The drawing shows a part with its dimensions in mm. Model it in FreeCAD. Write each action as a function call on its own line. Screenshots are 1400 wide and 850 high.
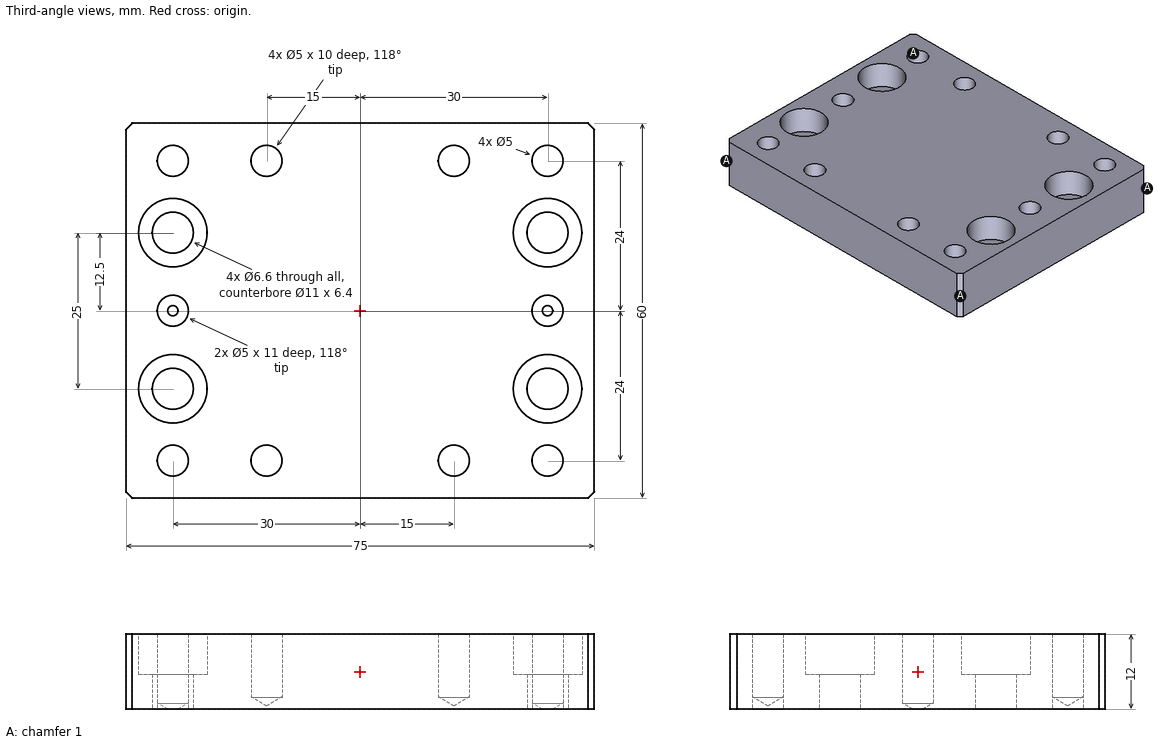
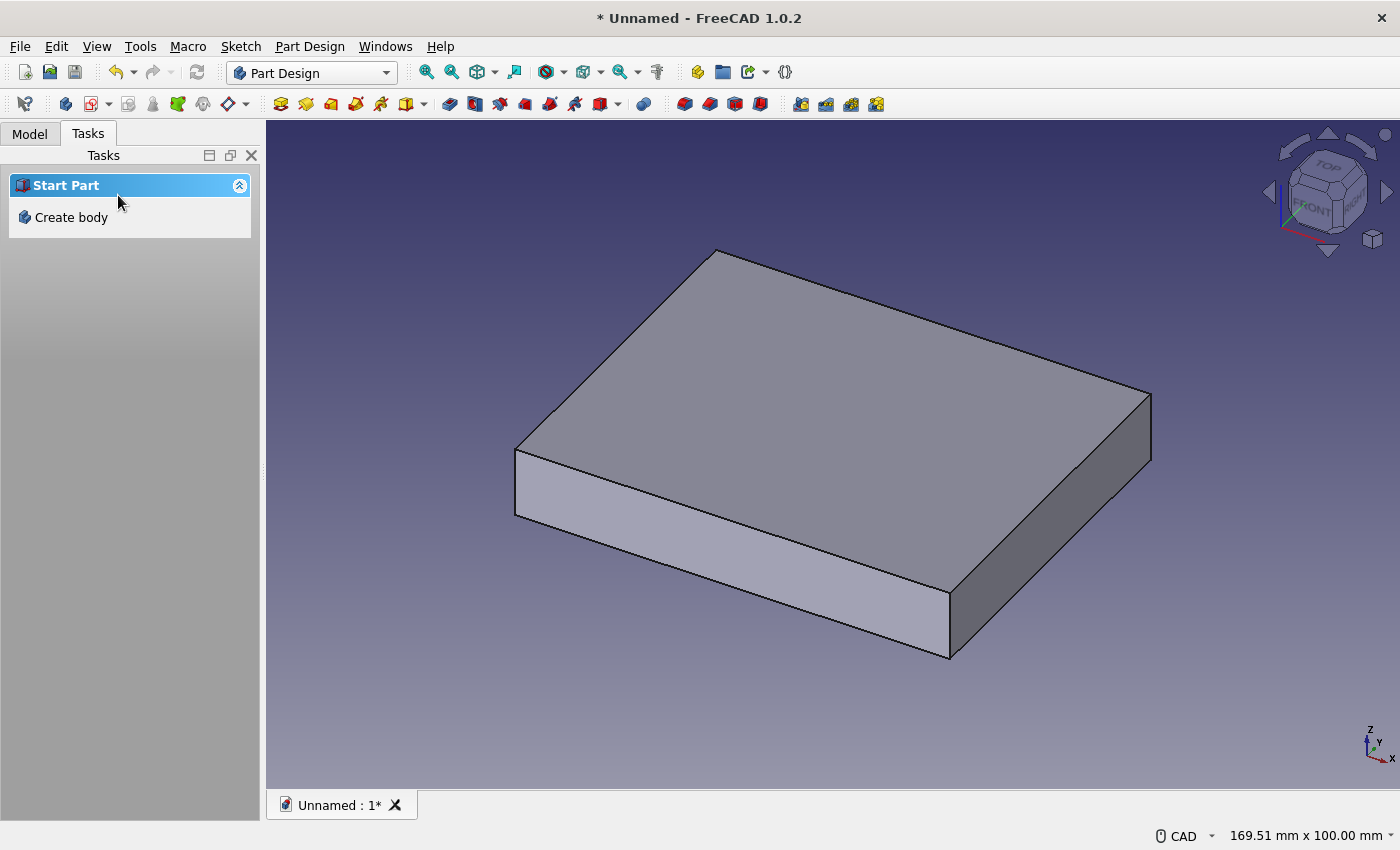
click(833, 421)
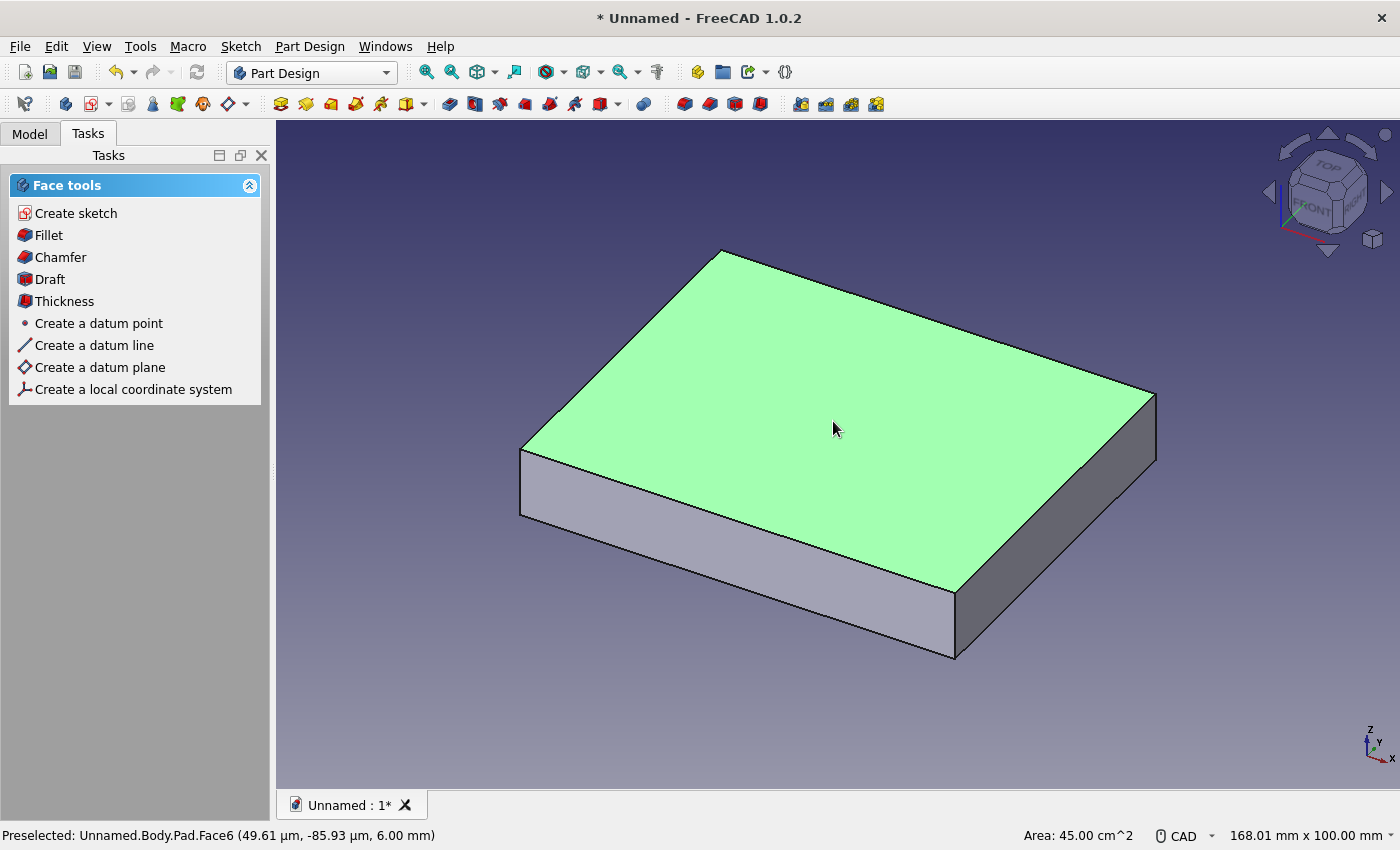
click(90, 104)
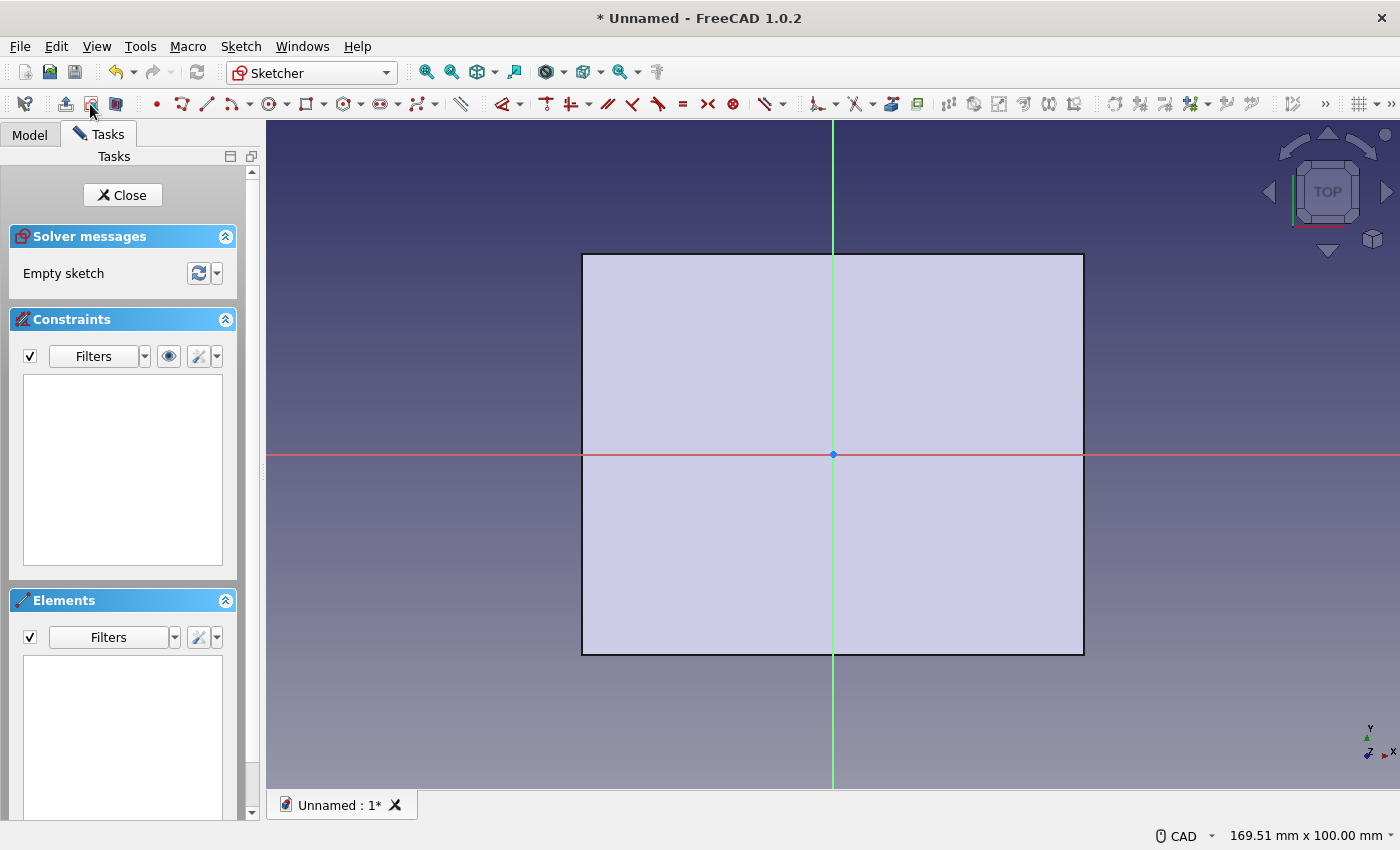
click(268, 104)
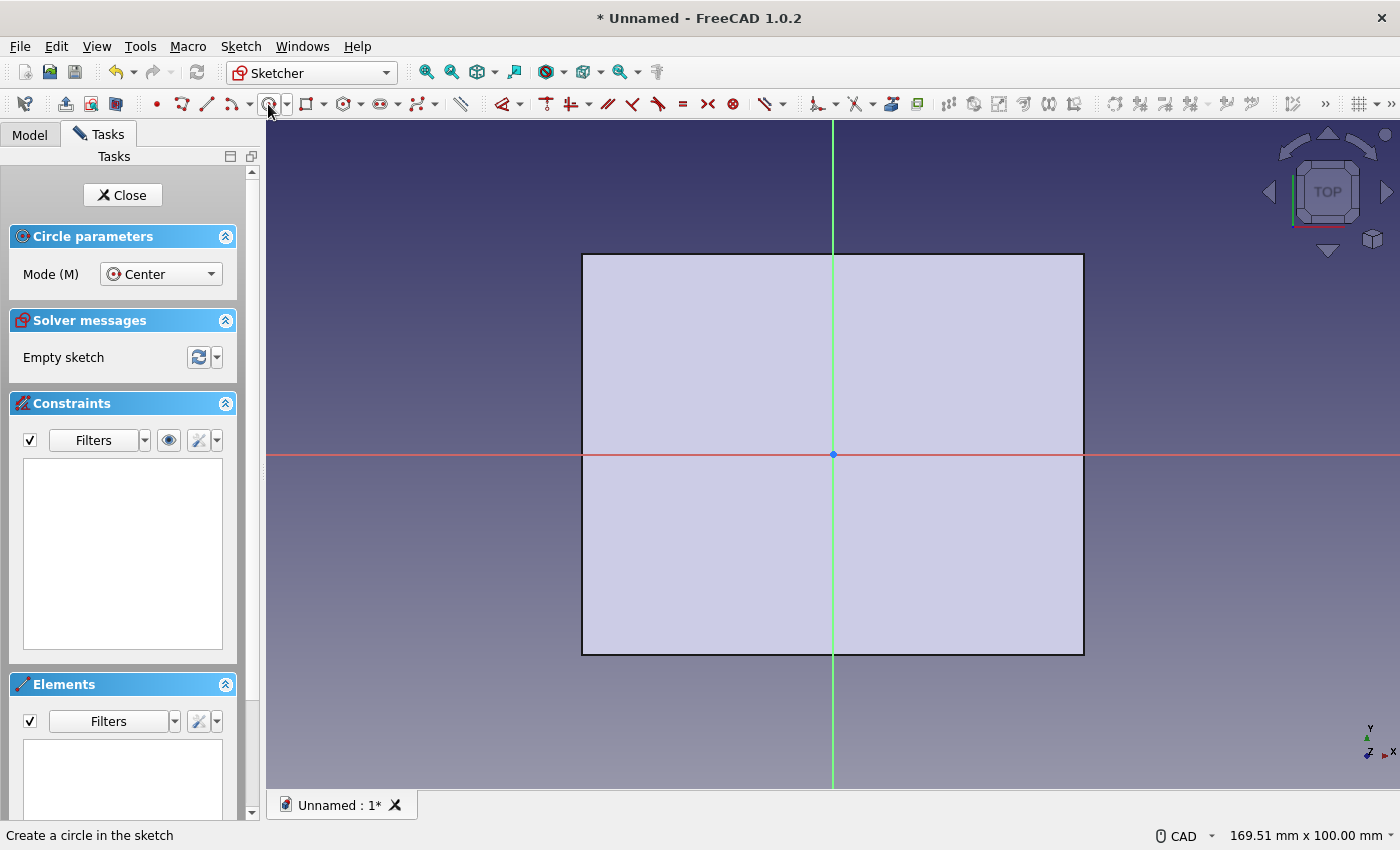
scroll(1034, 294, up, 2)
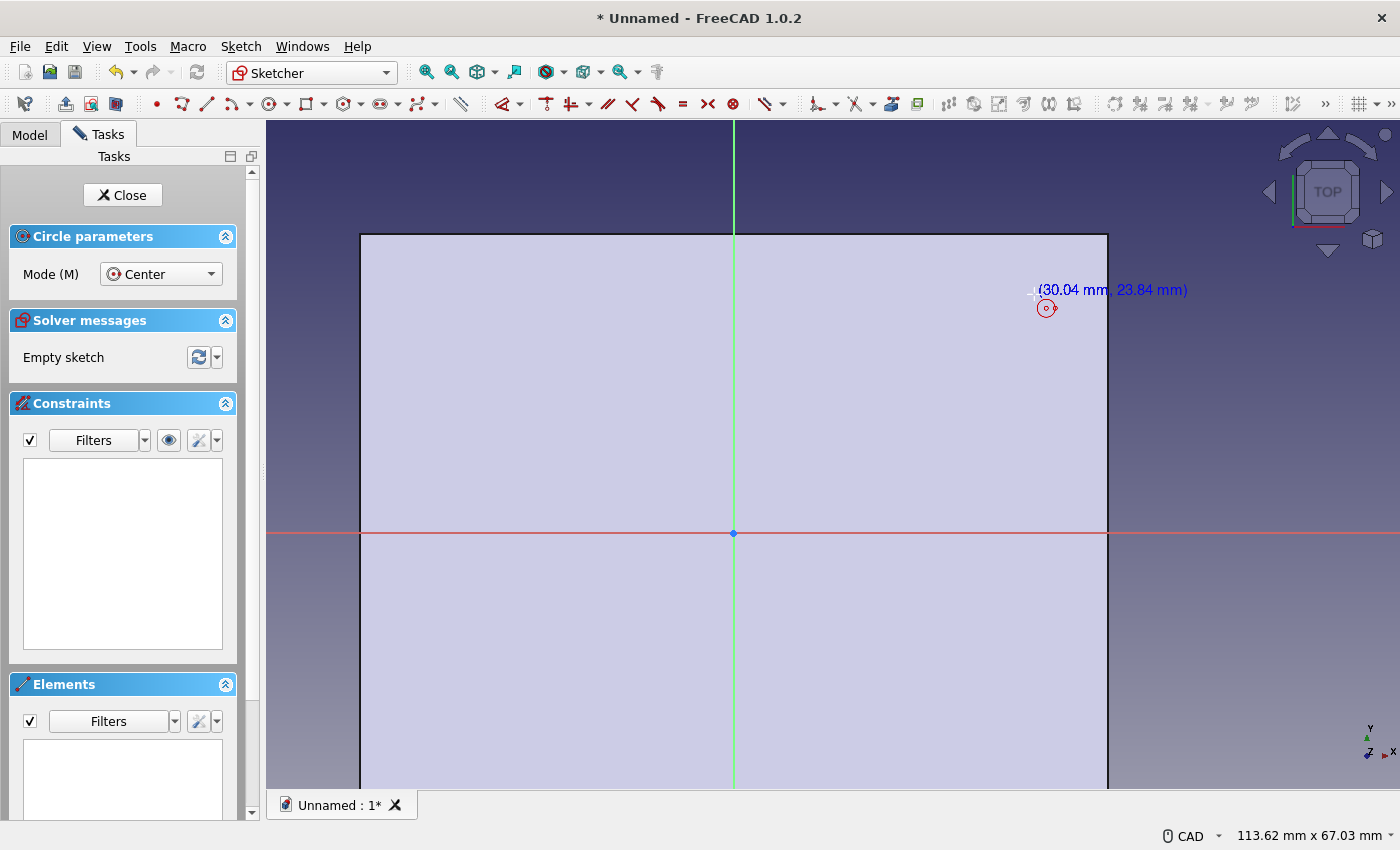
click(1033, 294)
click(1051, 276)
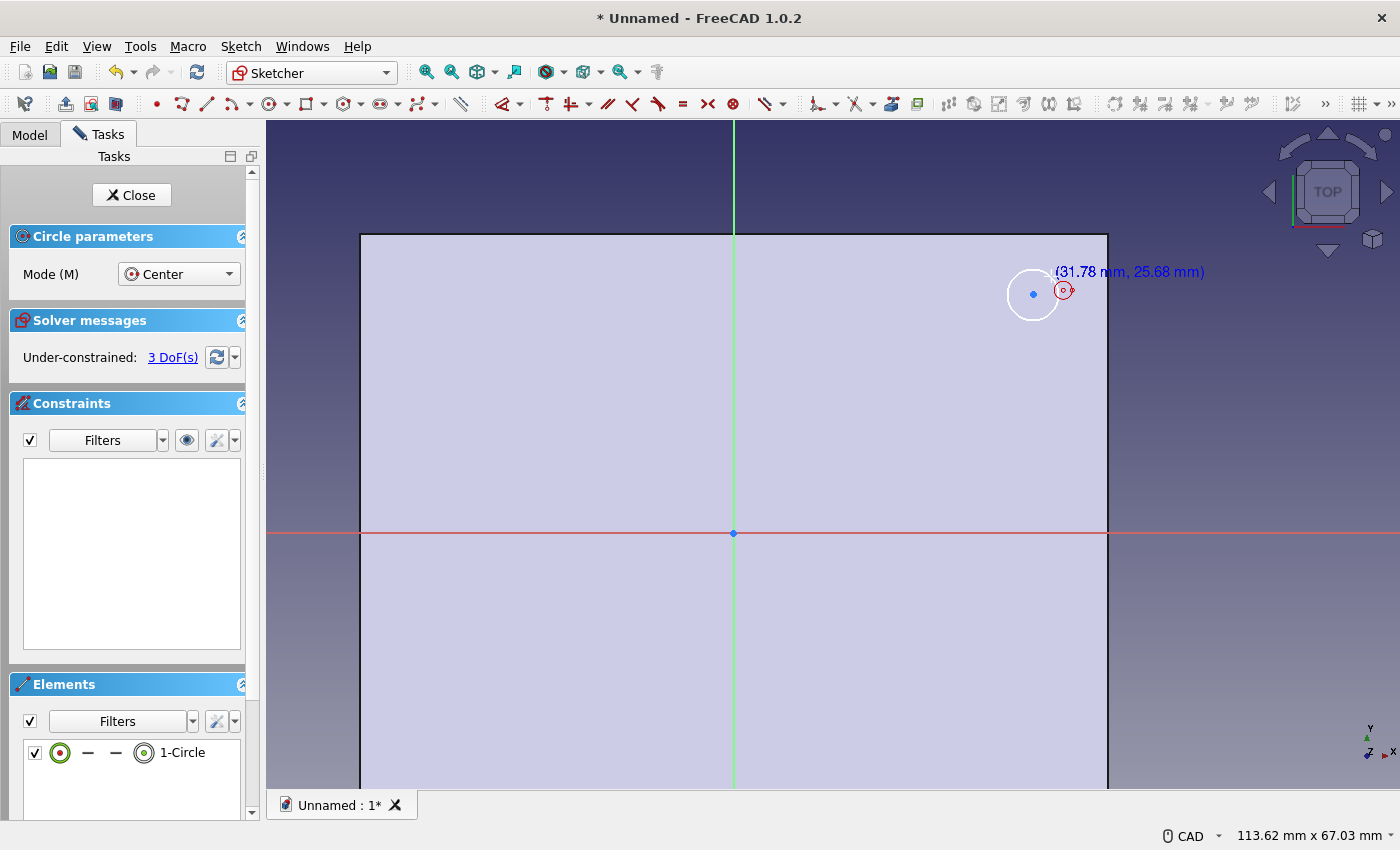
scroll(903, 148, down, 1)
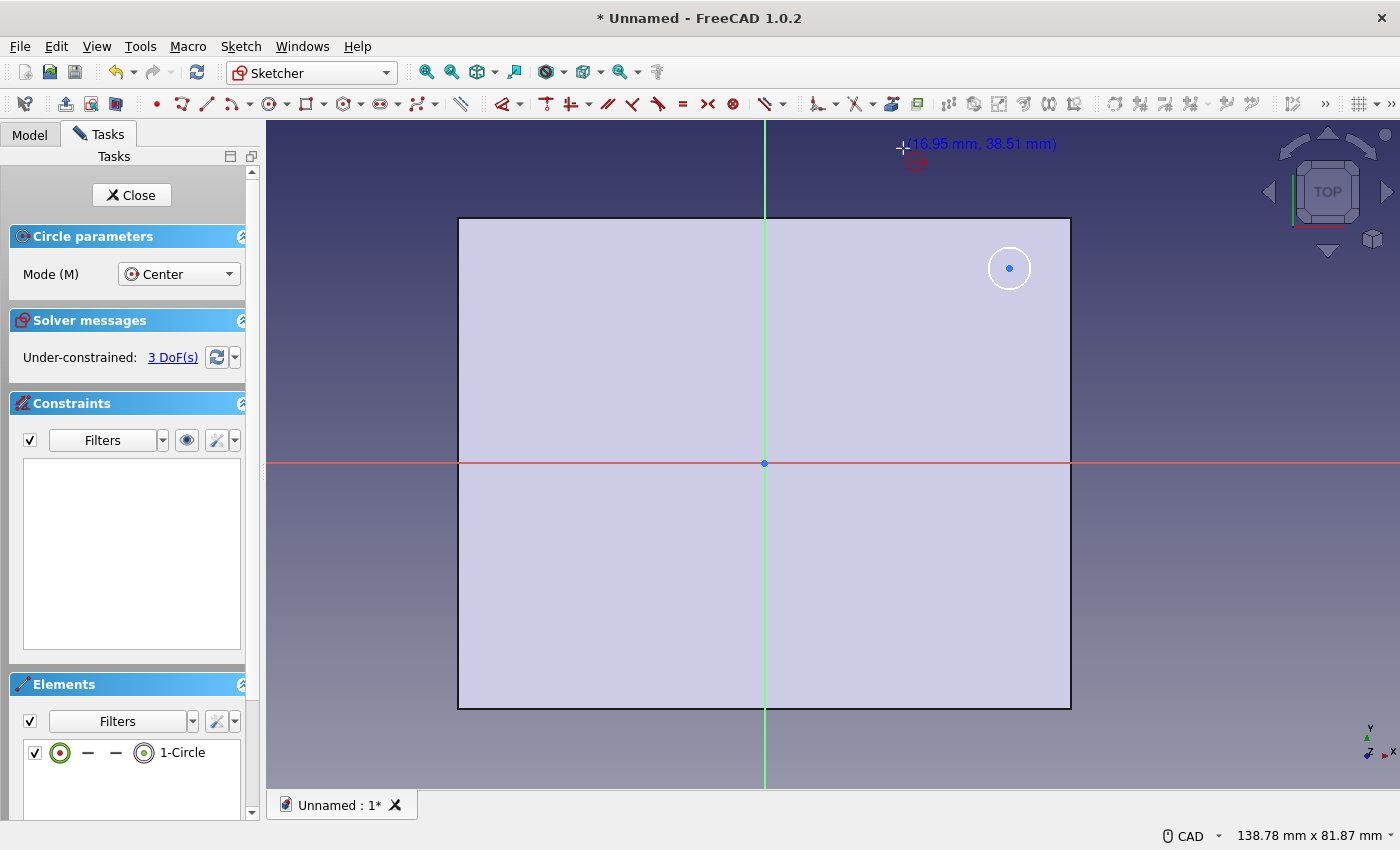
click(1010, 660)
click(1024, 645)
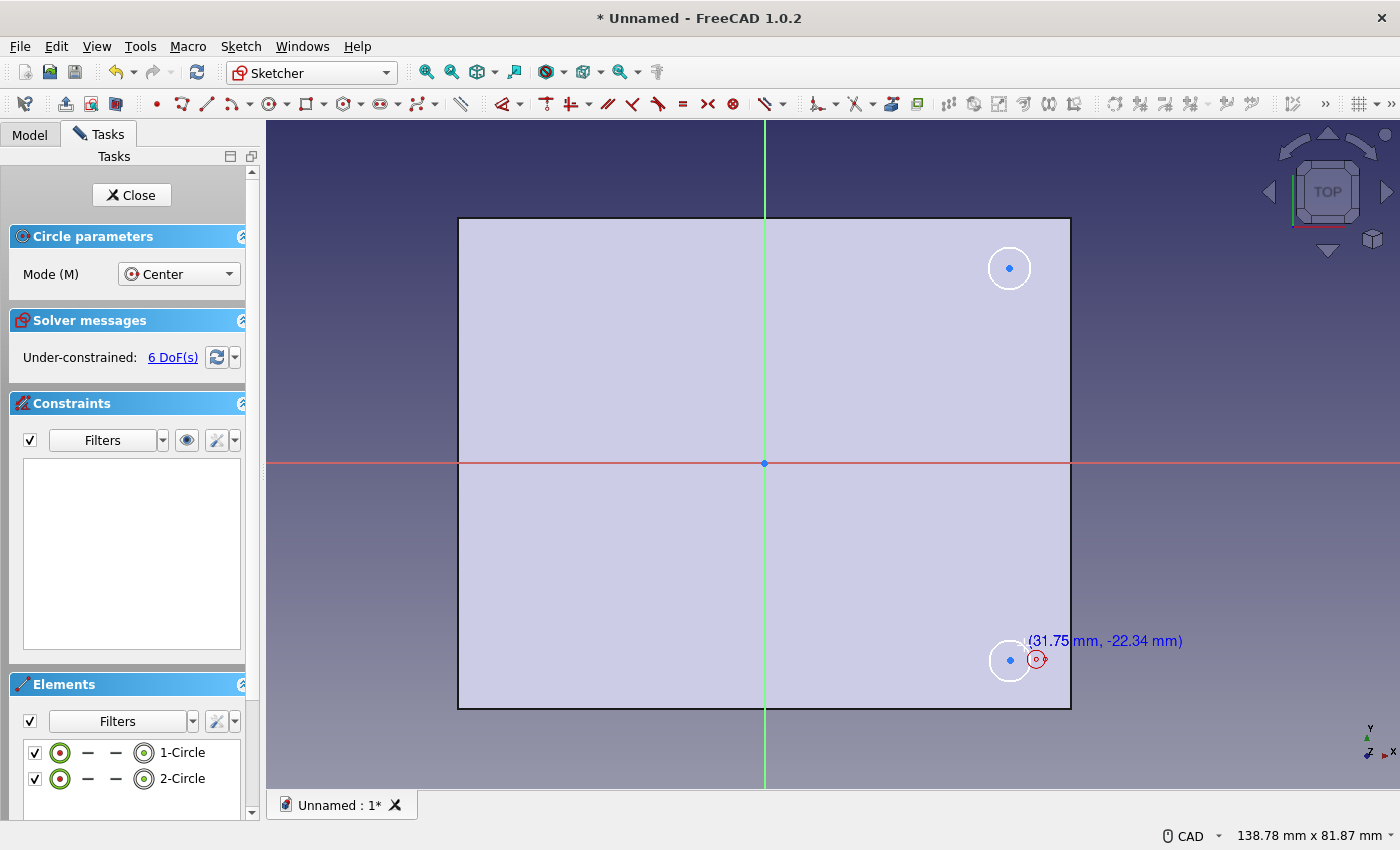
click(519, 660)
click(534, 645)